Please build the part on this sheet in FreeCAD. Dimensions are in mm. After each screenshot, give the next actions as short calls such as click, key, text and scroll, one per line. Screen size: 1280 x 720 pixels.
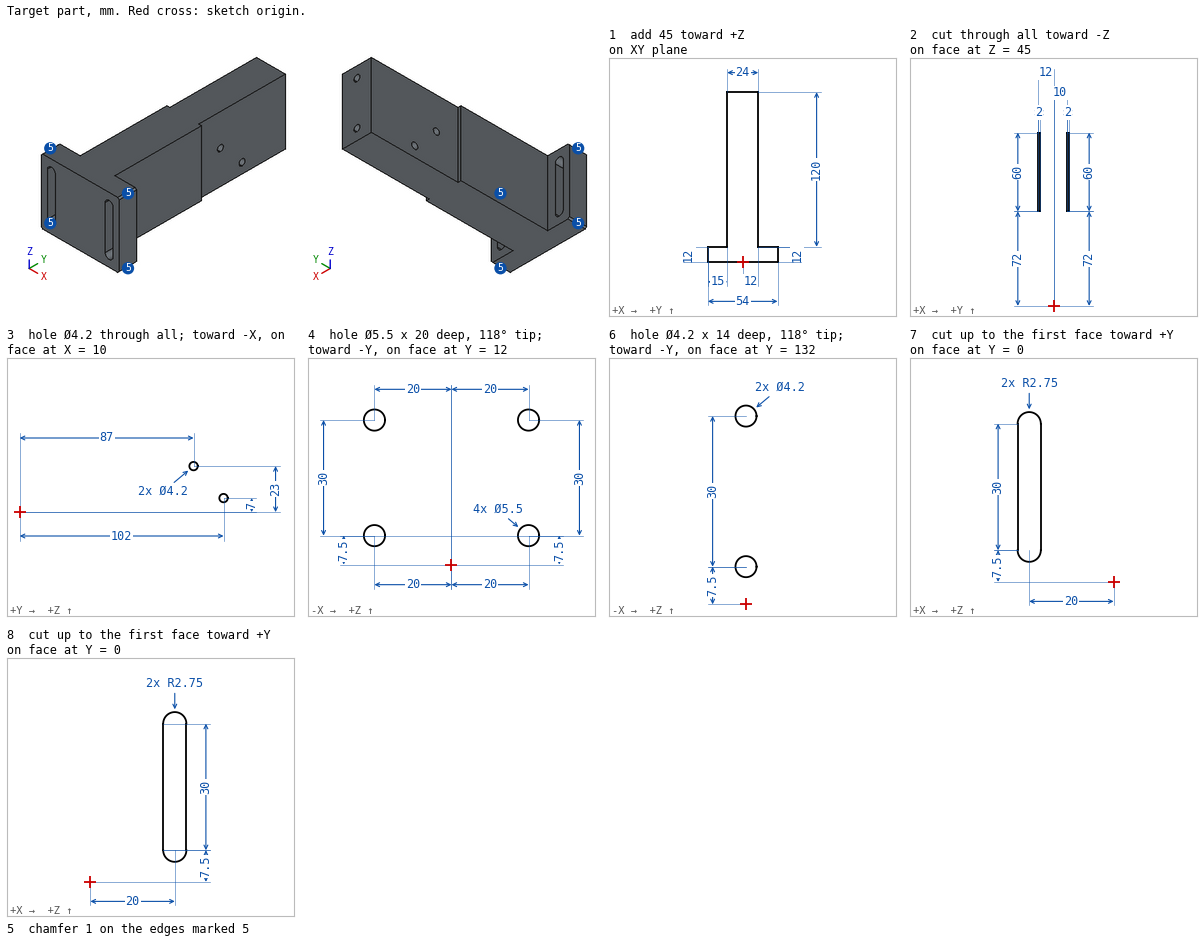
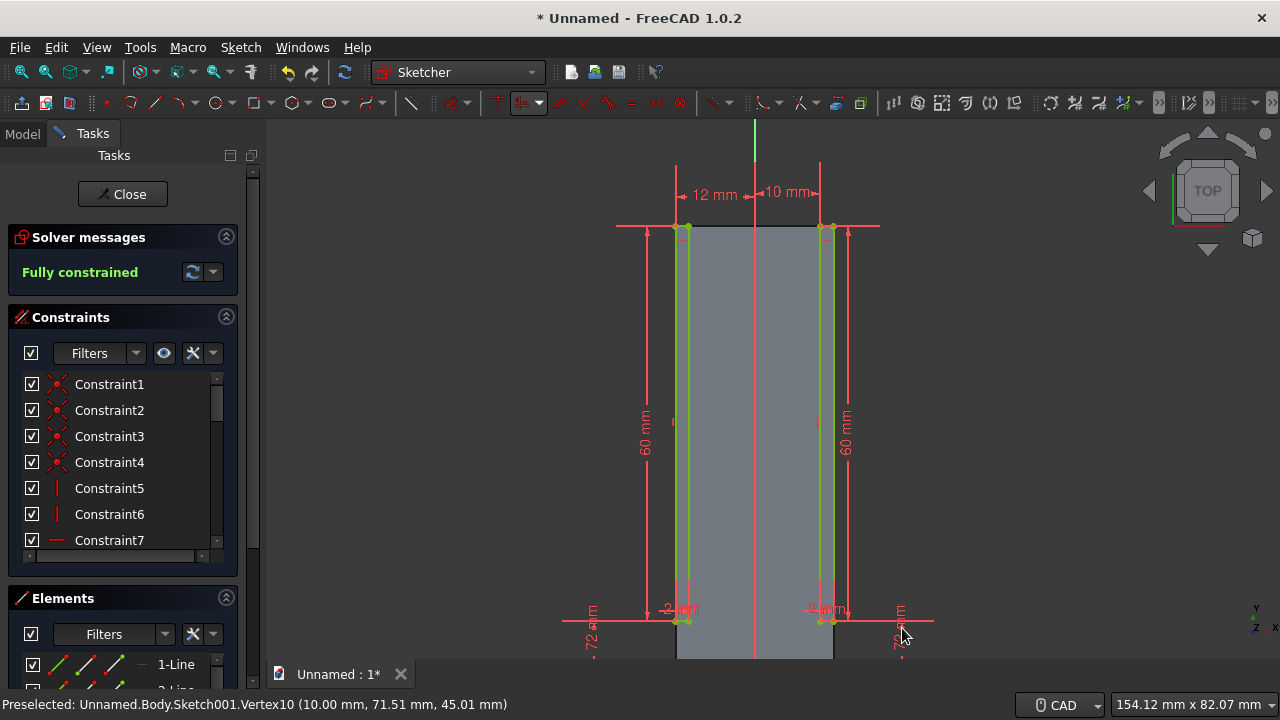
click(123, 194)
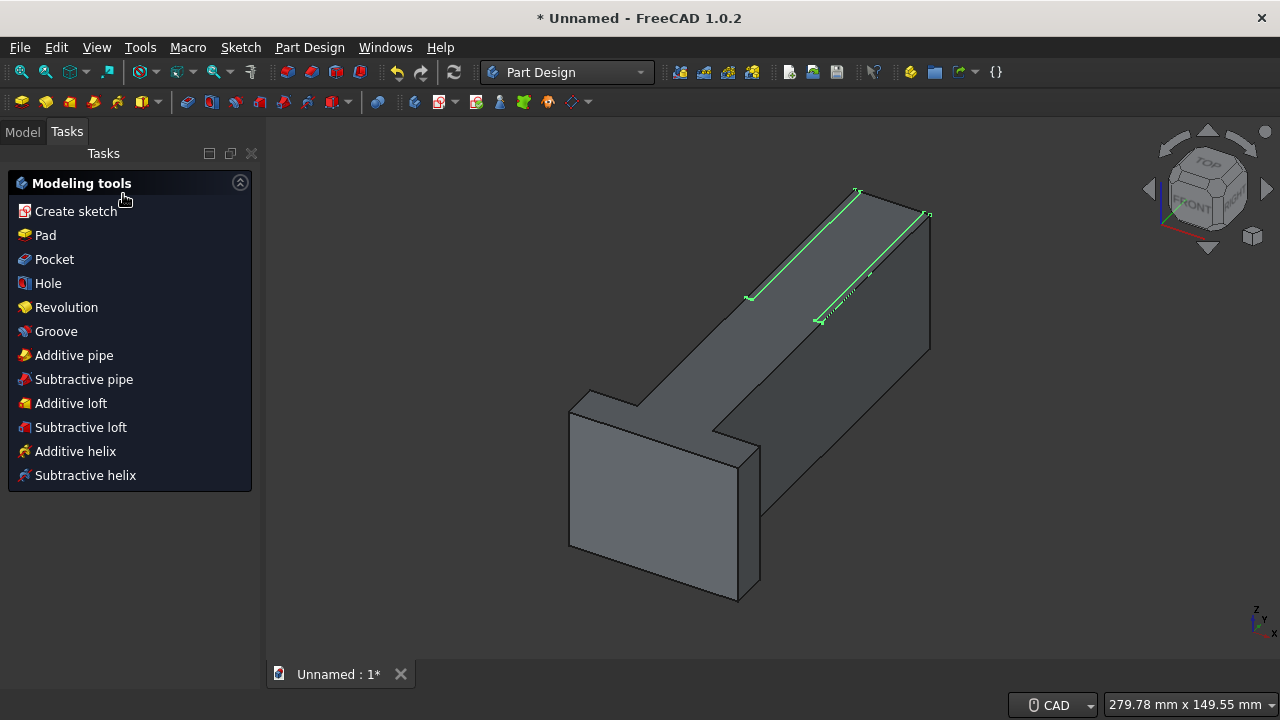
click(188, 102)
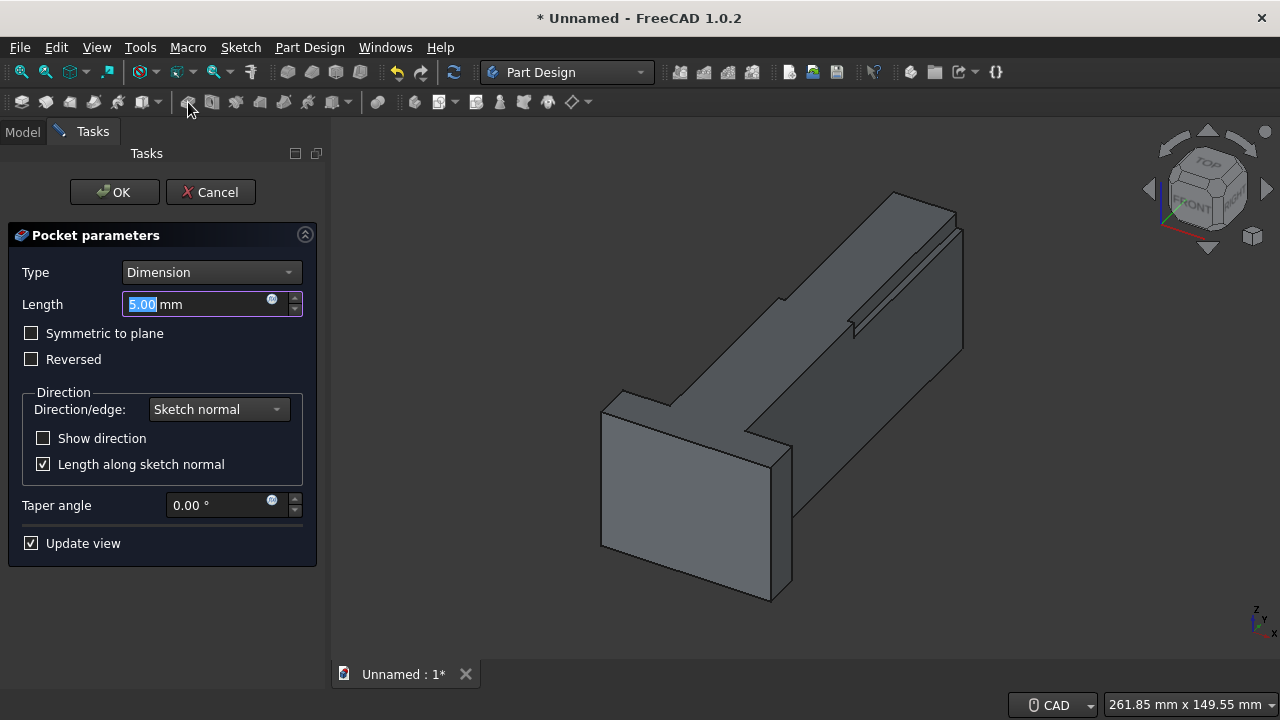
click(212, 272)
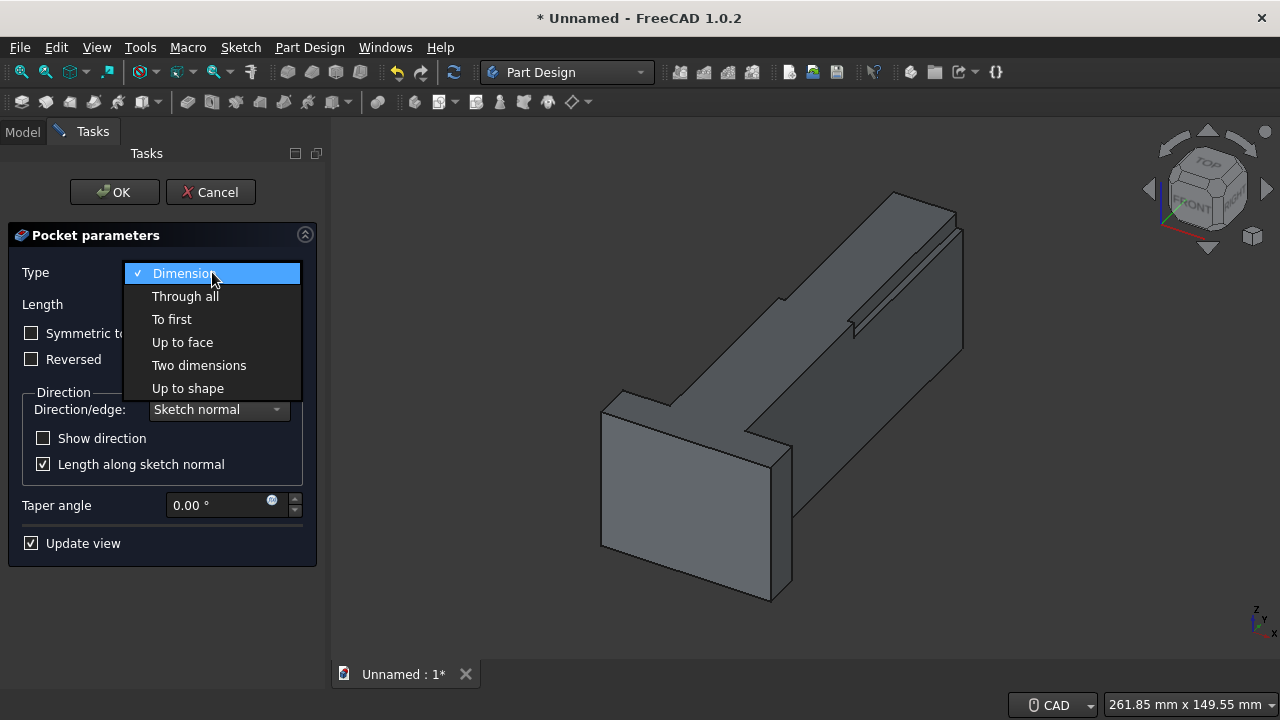
click(212, 296)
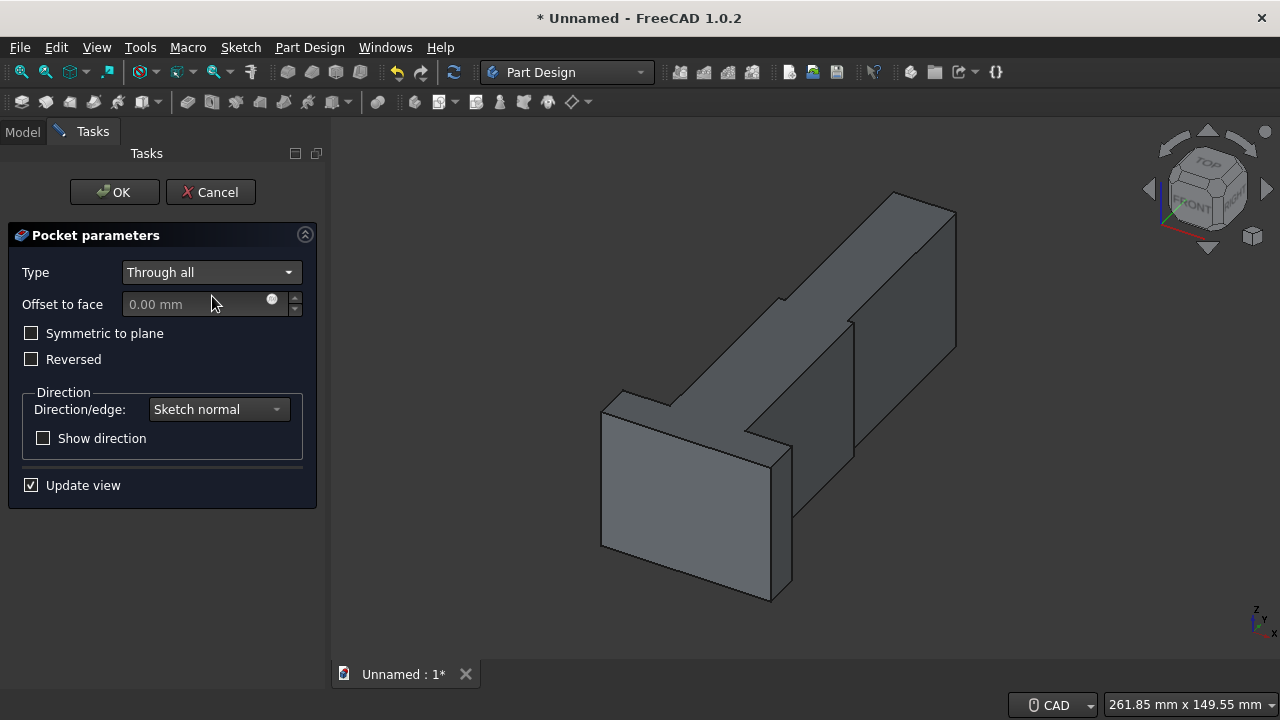
click(115, 192)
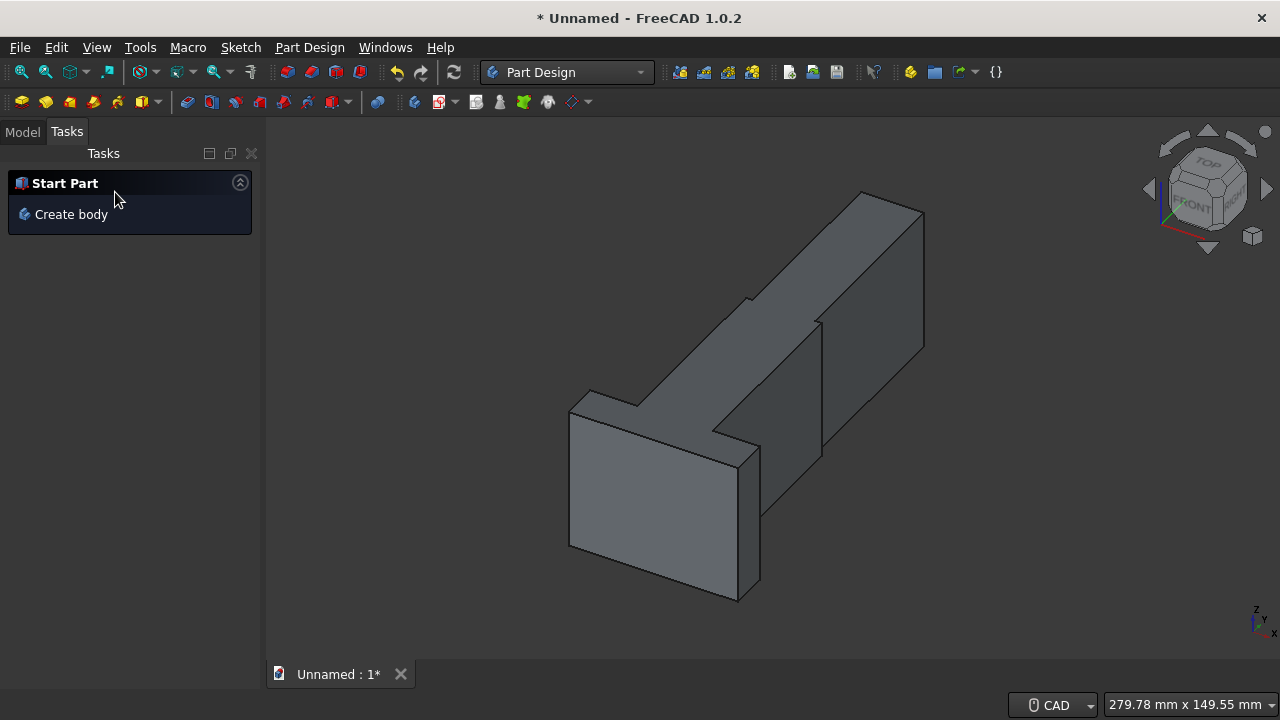
click(870, 333)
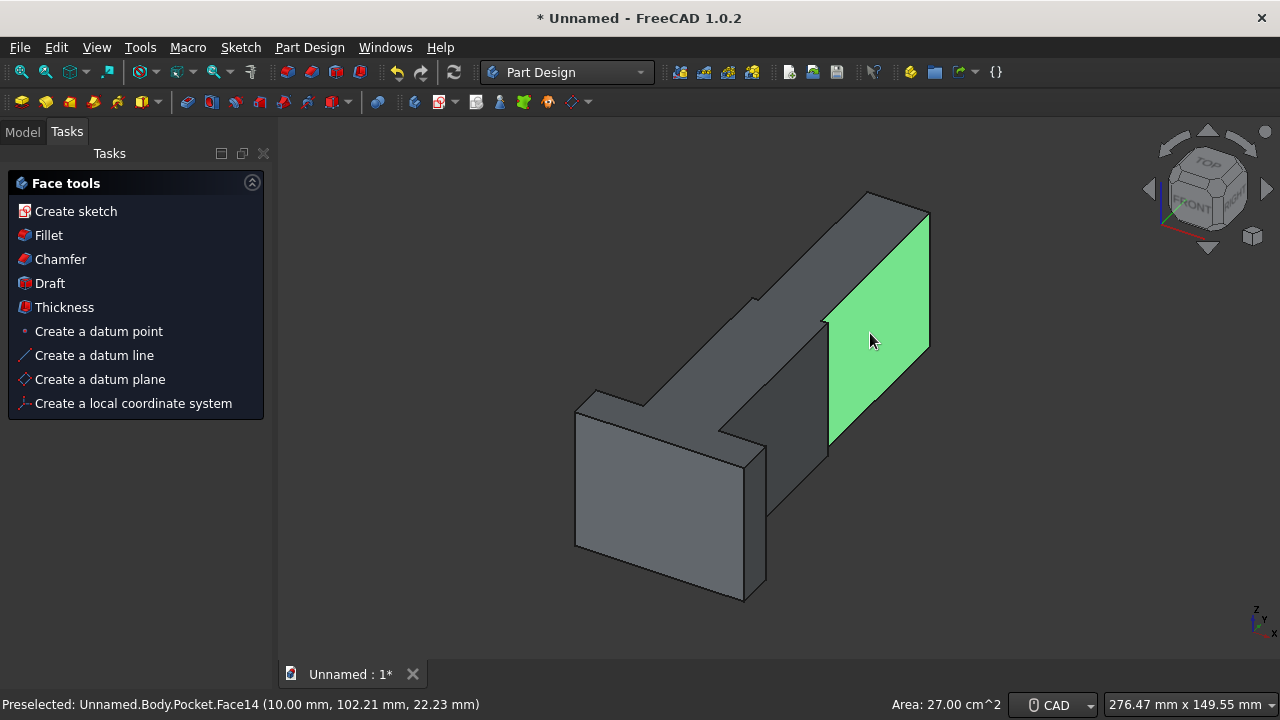
click(440, 102)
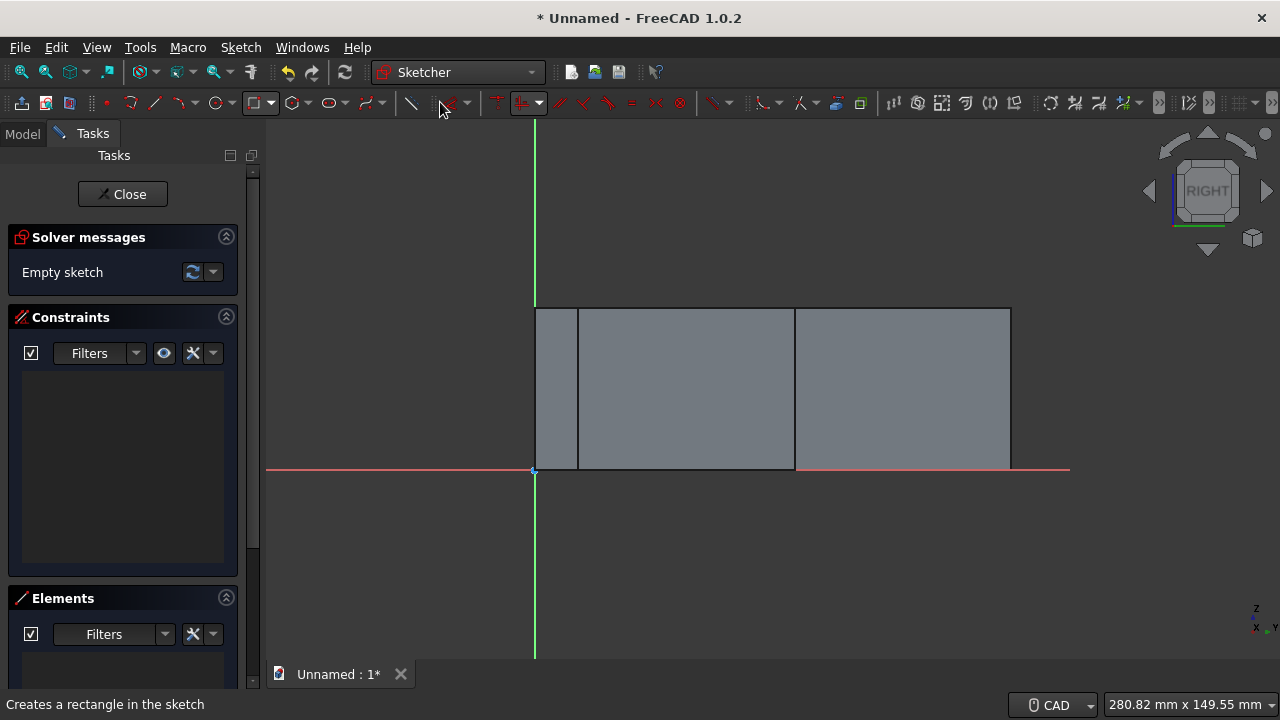
click(70, 104)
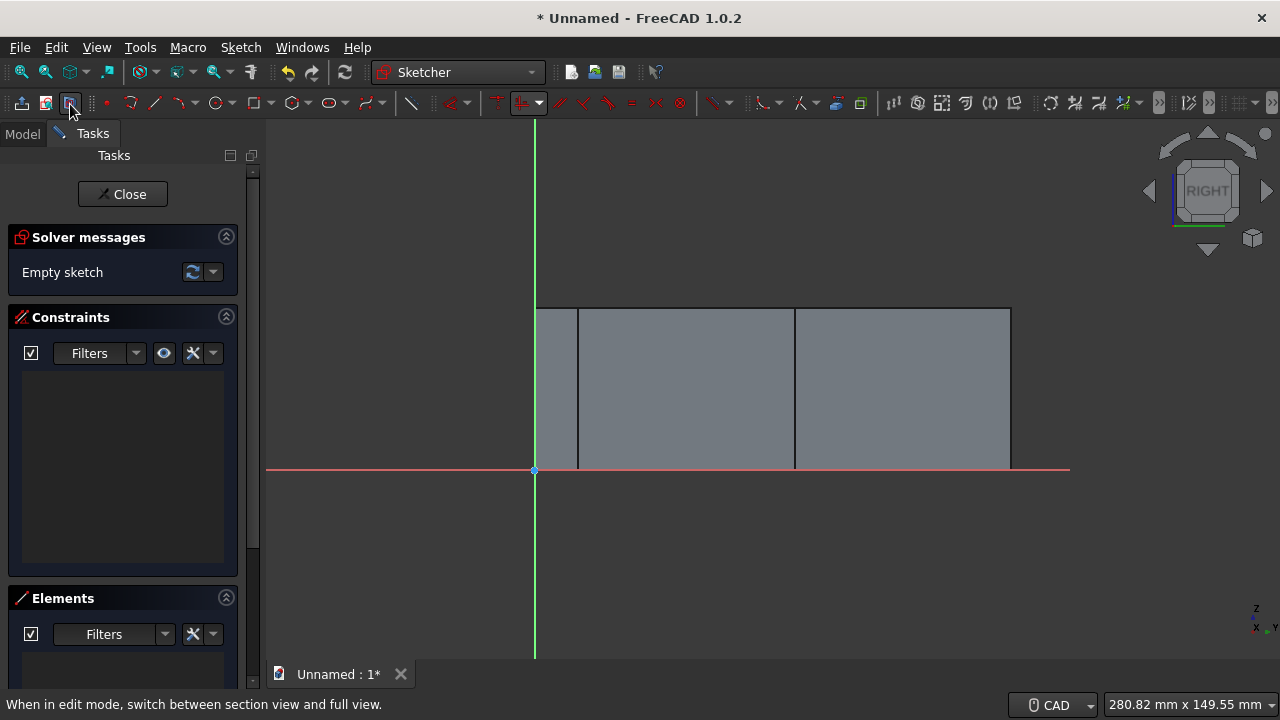
scroll(919, 423, up, 8)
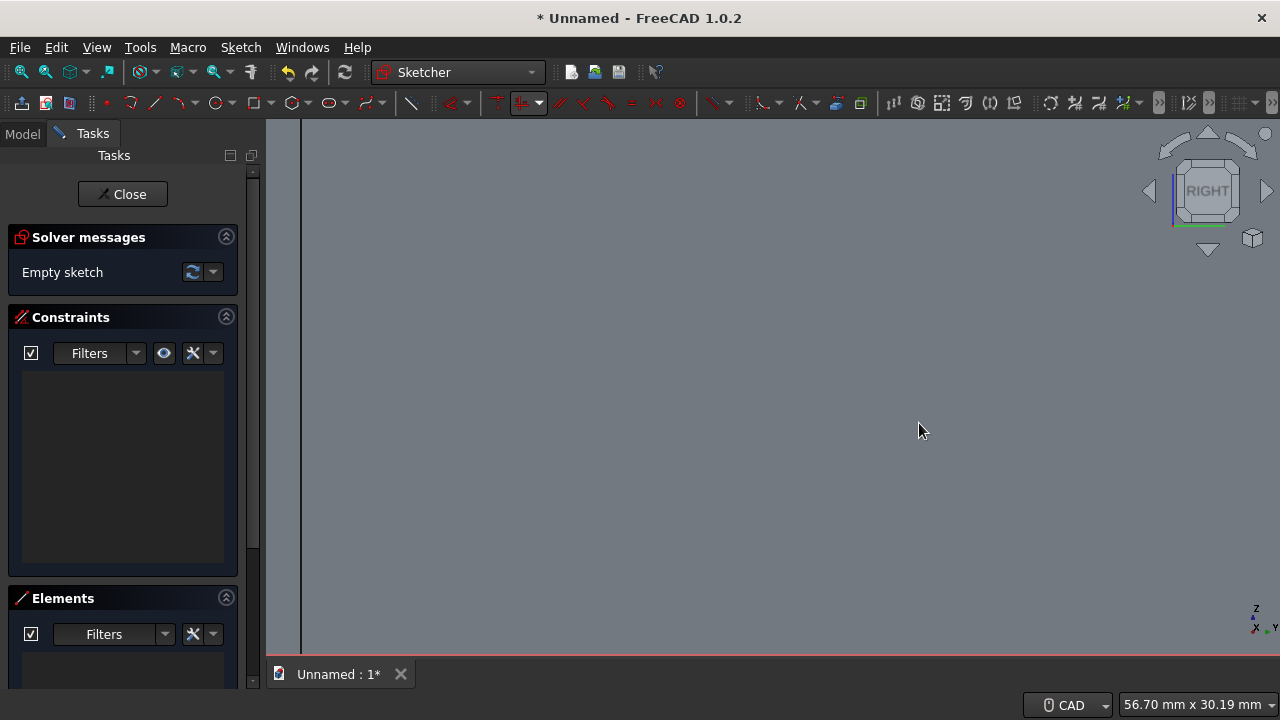
click(216, 104)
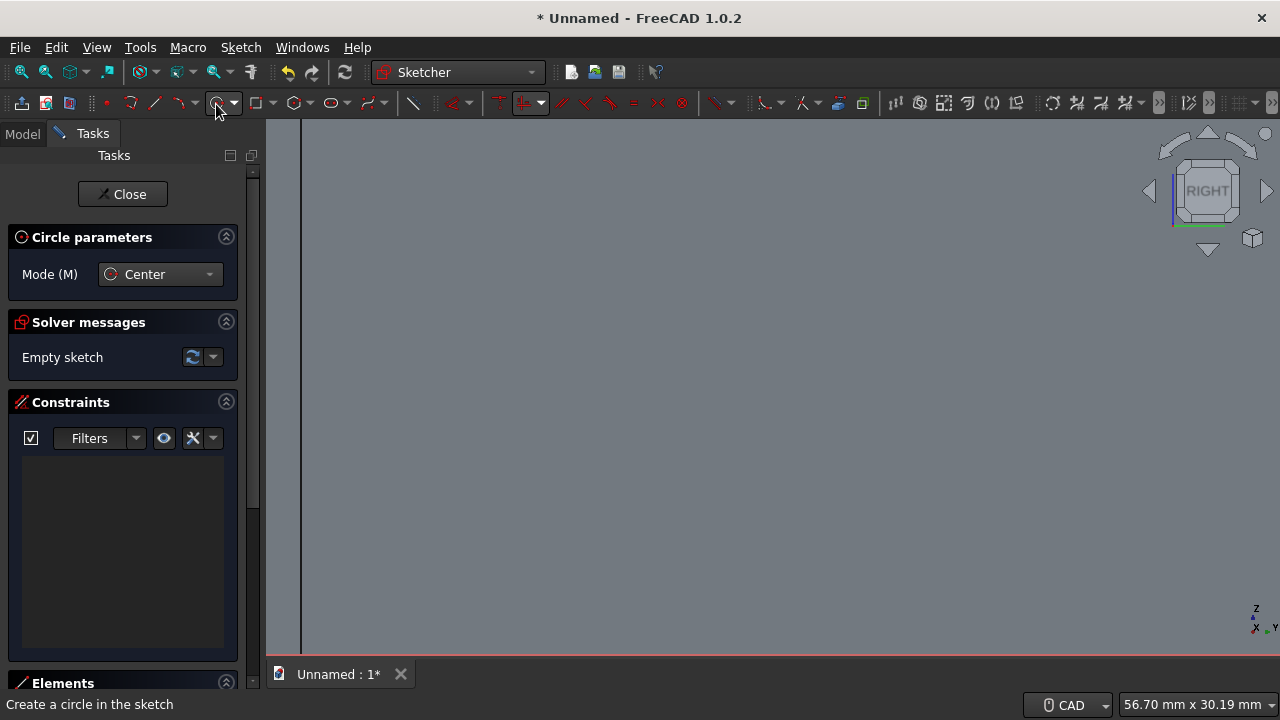
click(837, 530)
move(864, 503)